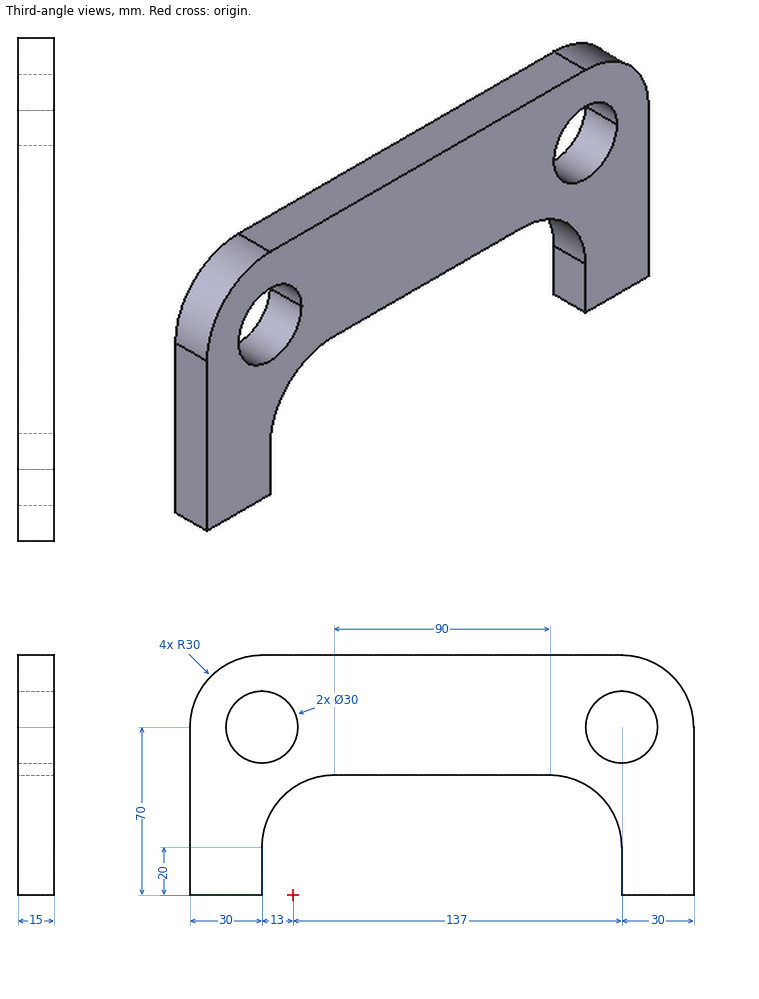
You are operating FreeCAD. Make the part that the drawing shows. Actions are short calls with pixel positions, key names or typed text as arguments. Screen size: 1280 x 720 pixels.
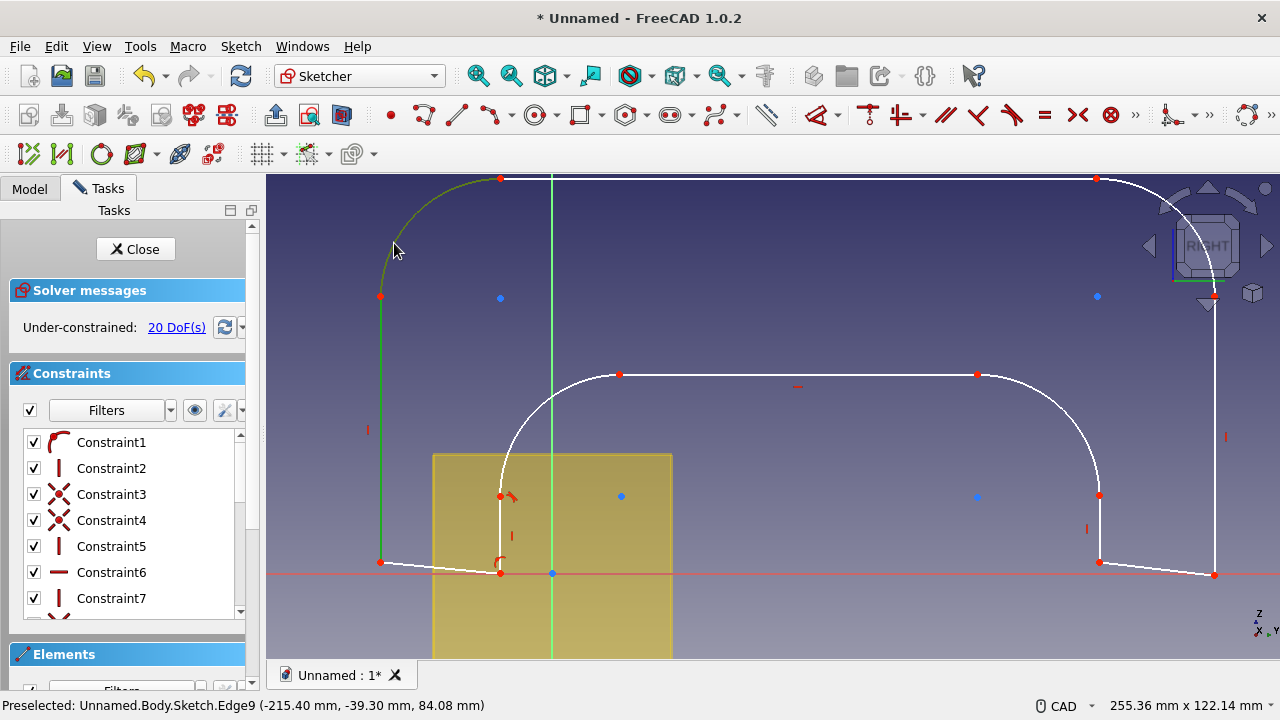
click(1012, 116)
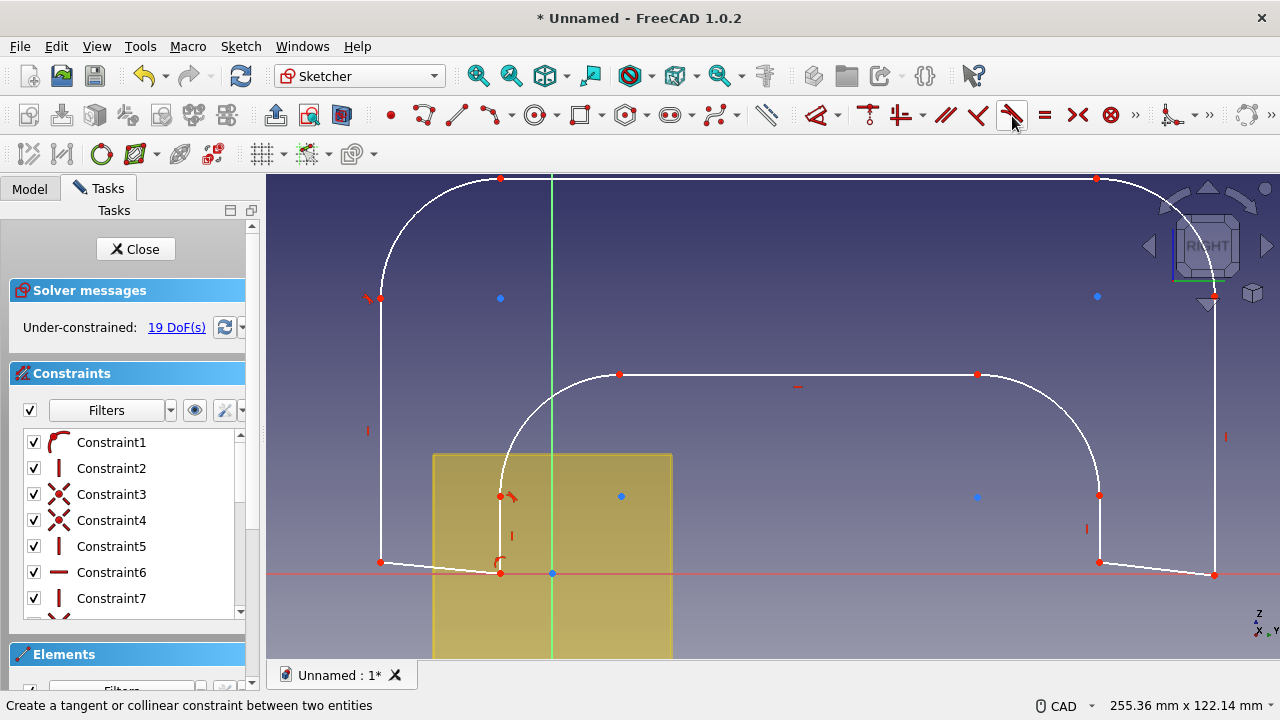
scroll(513, 500, down, 2)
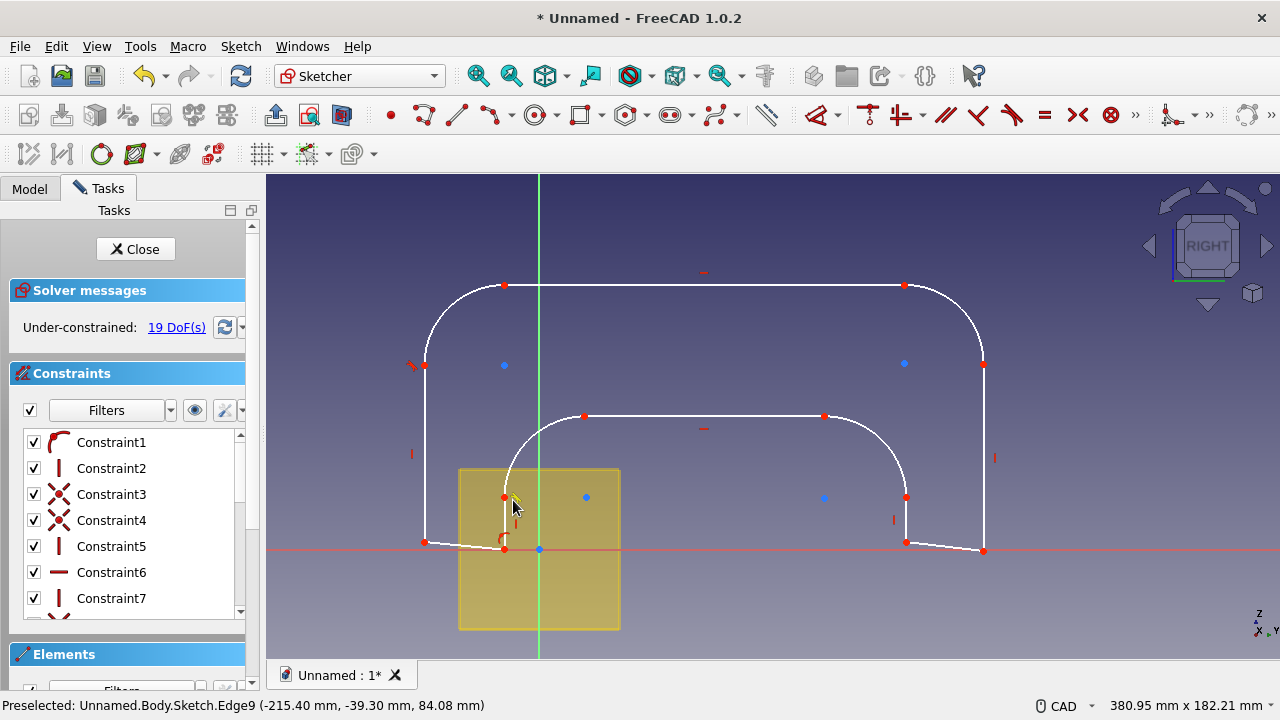
click(625, 285)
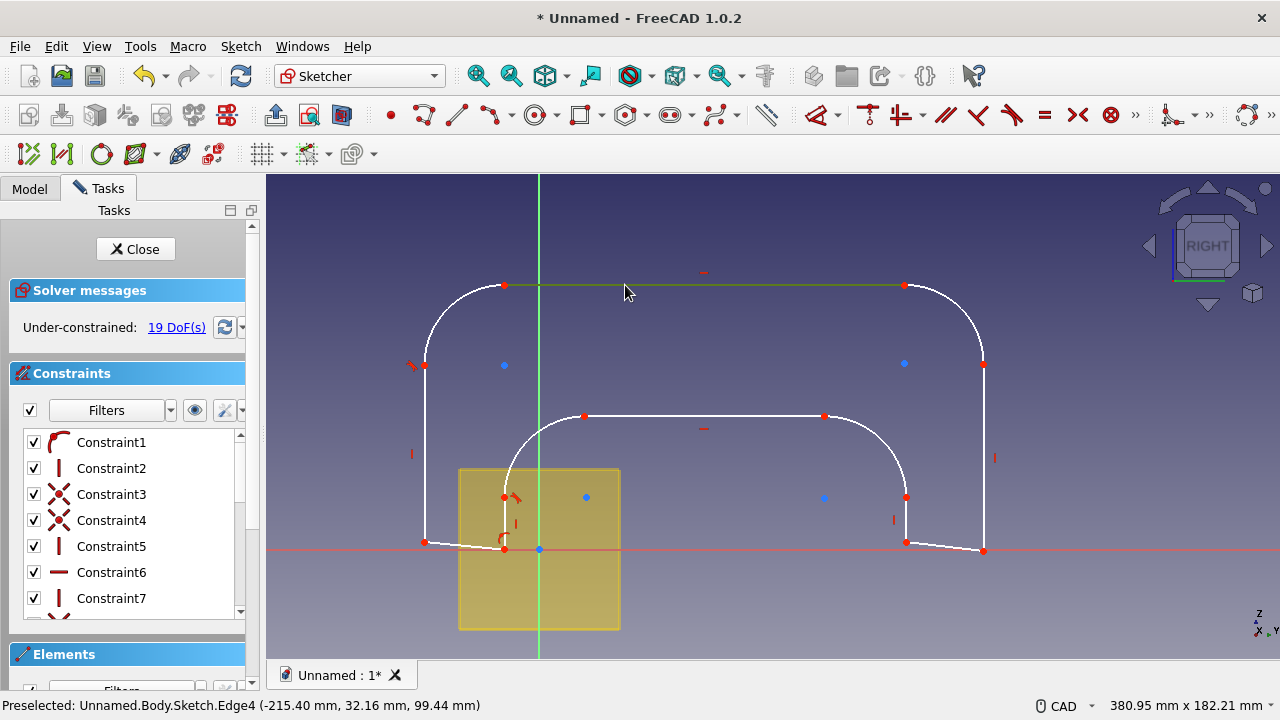
click(468, 294)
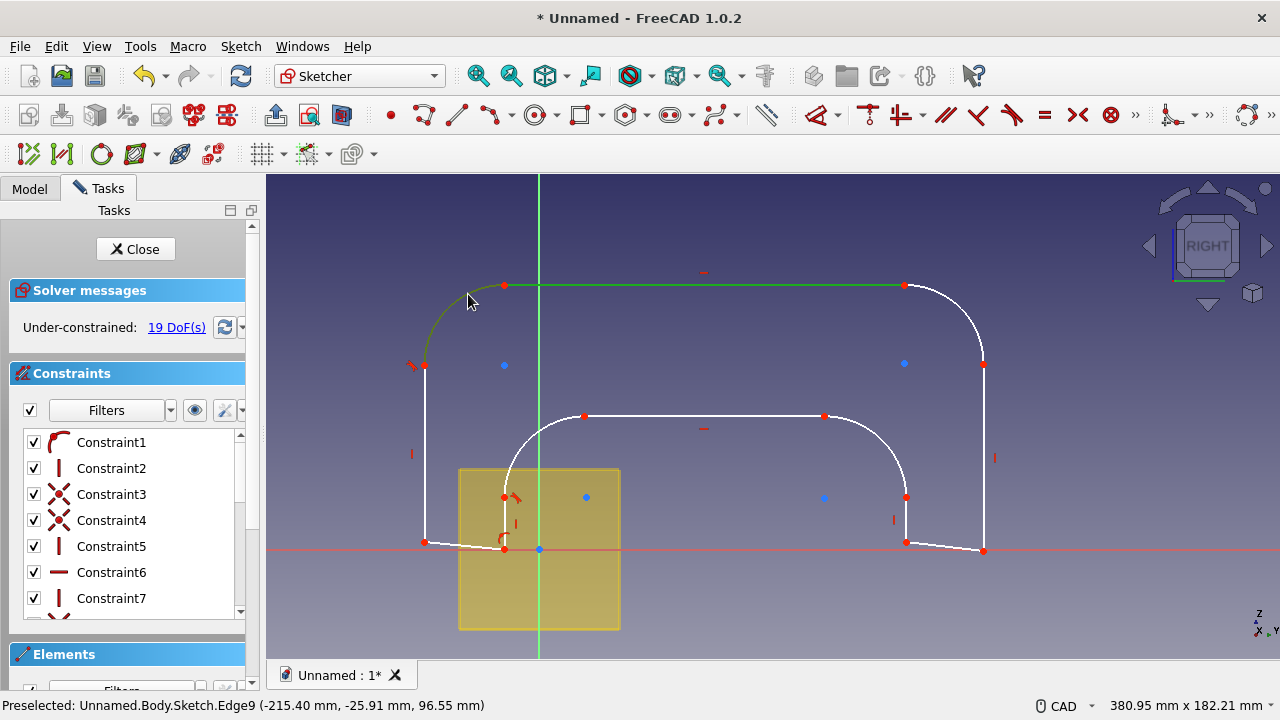
click(1012, 116)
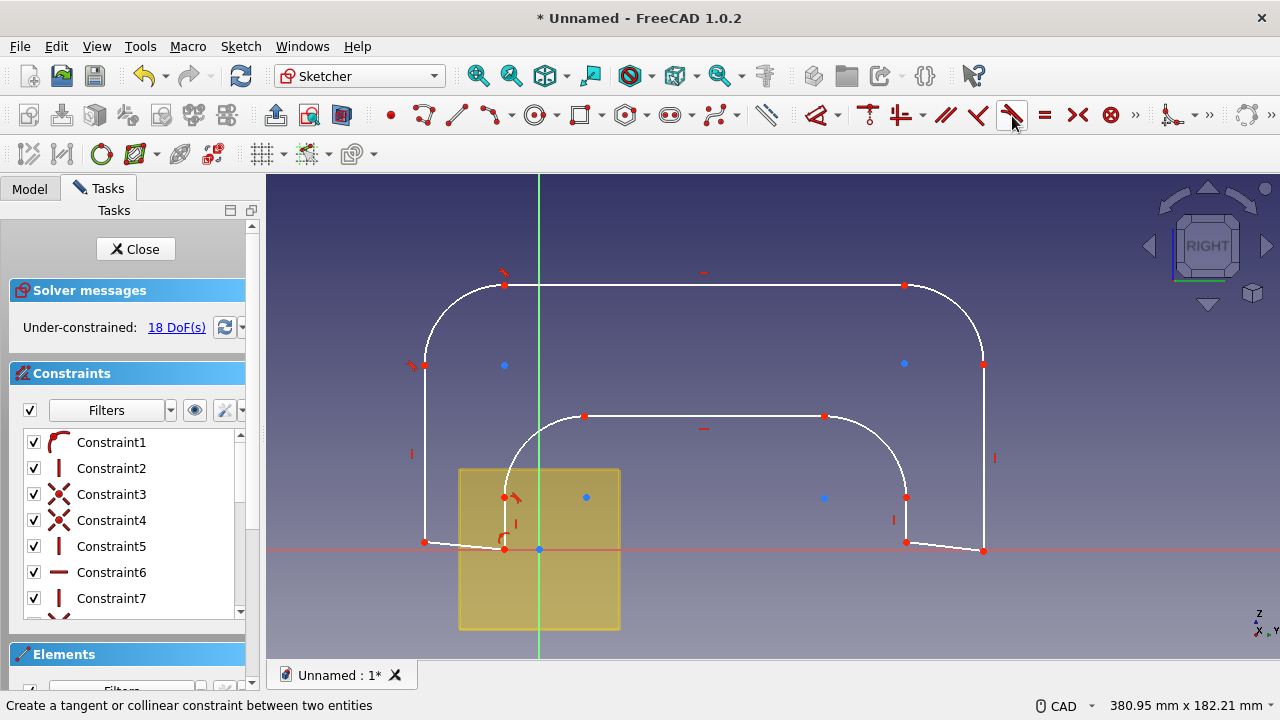
click(625, 285)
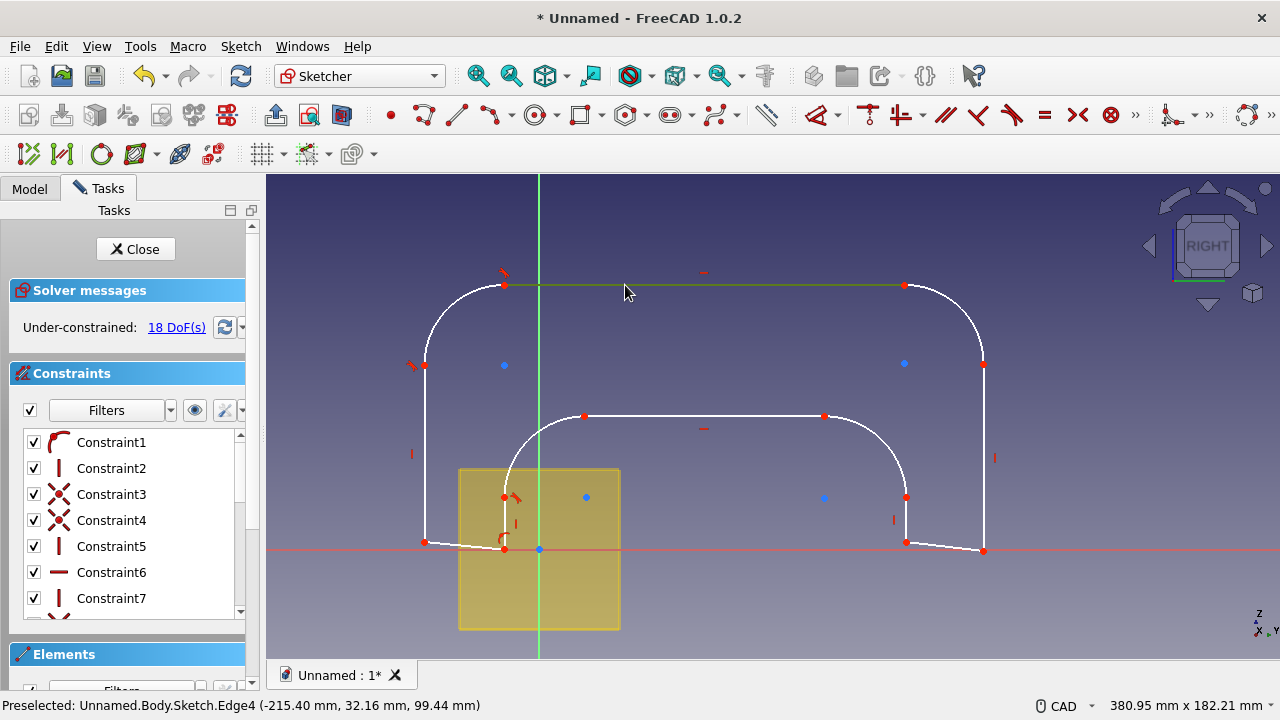
click(975, 328)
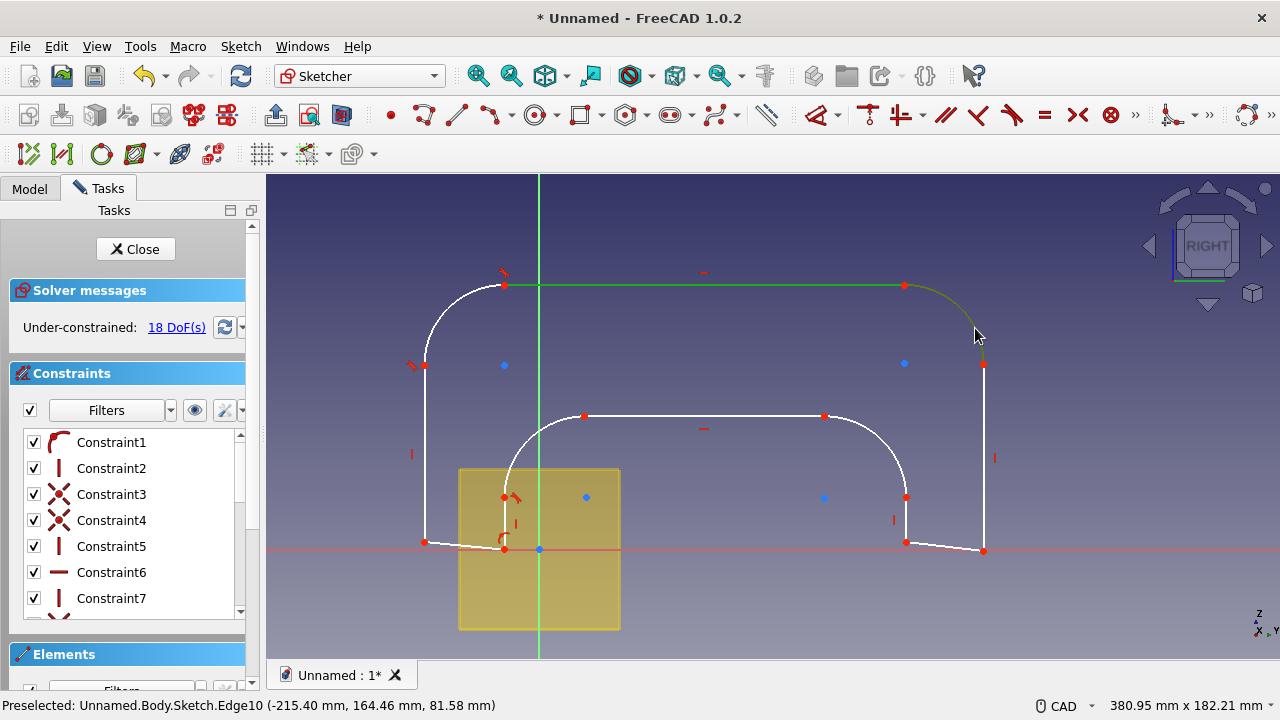
key(t)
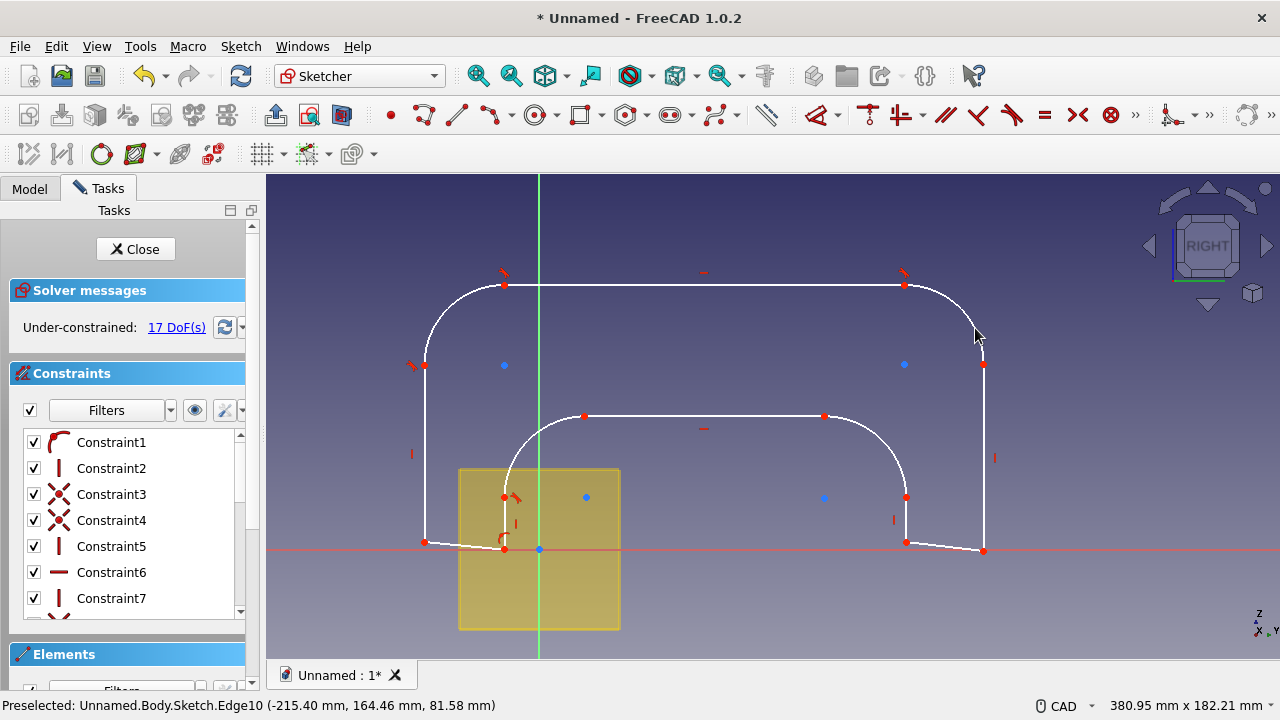
click(984, 420)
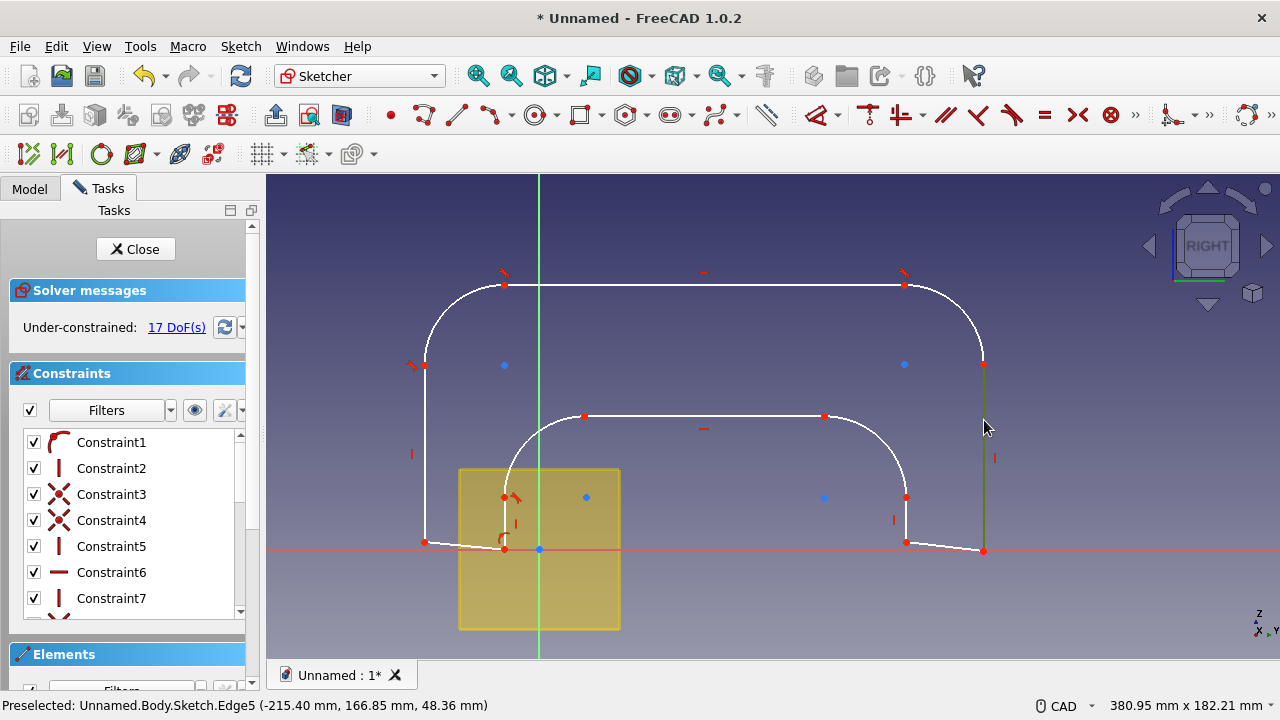
click(975, 328)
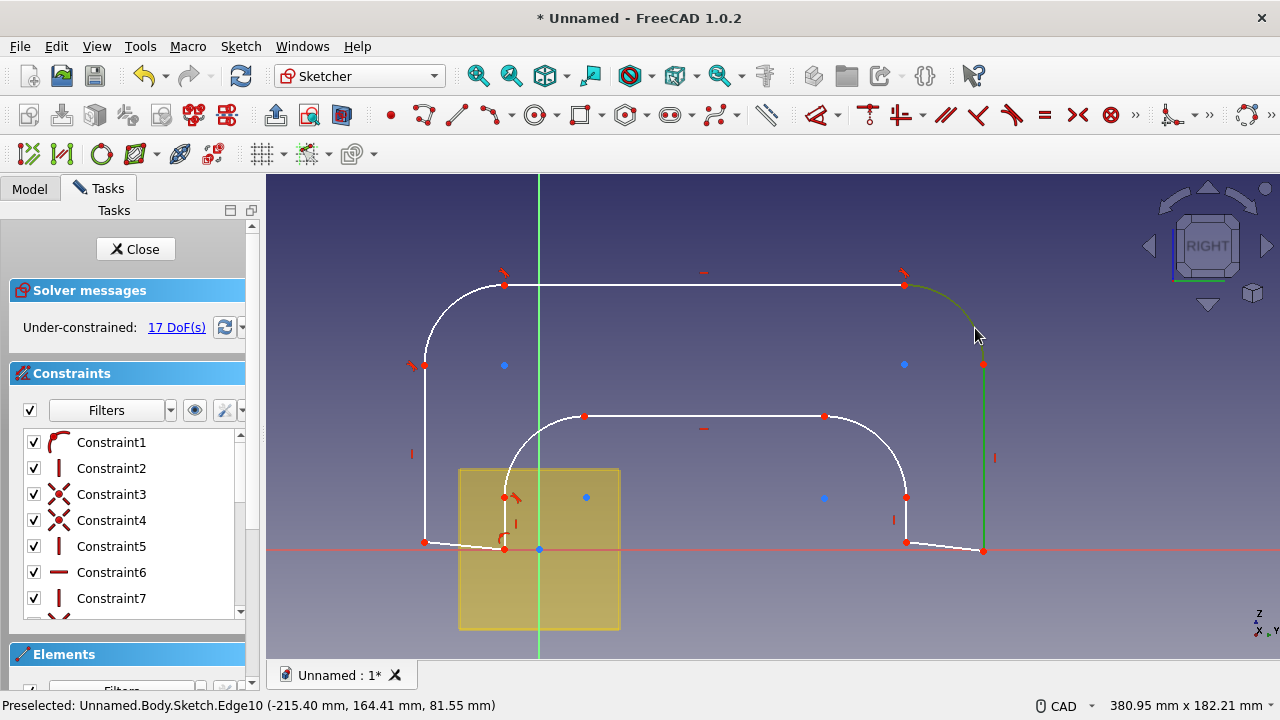
key(t)